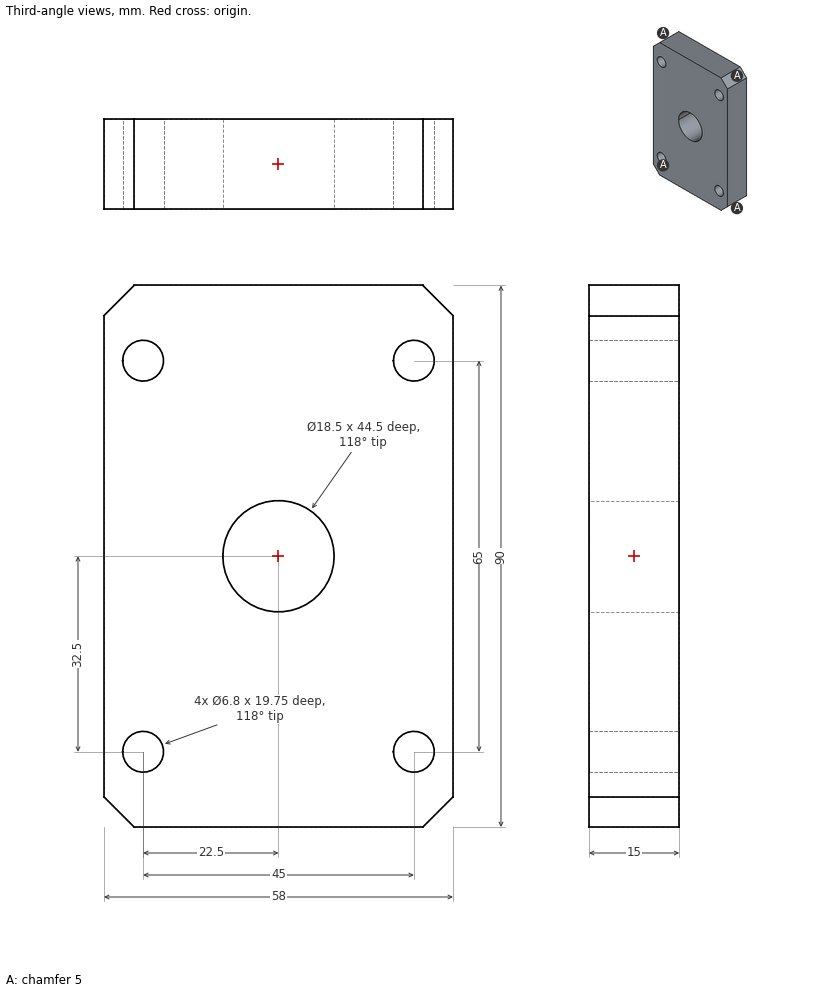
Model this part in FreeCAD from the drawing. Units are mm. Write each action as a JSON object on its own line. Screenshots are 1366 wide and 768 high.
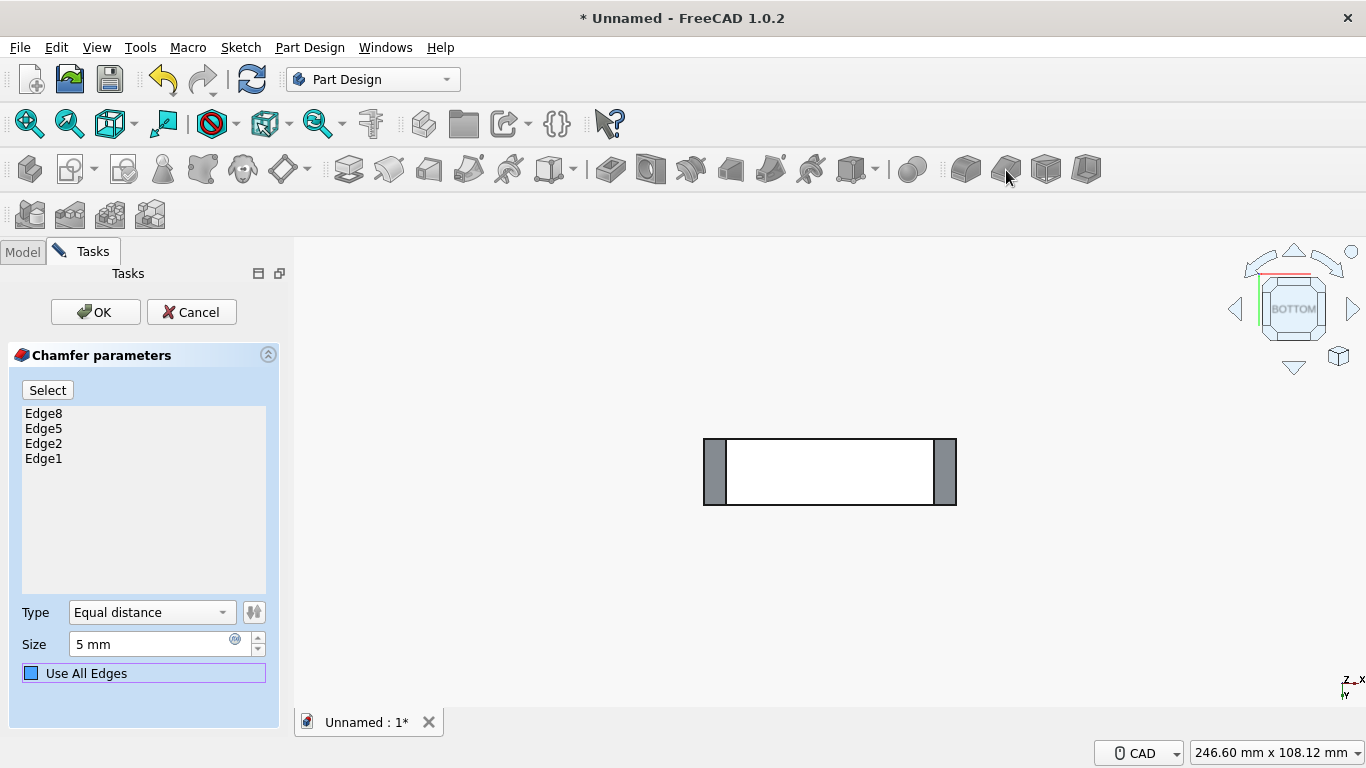
{"action": "left_click", "coordinate": [96, 312]}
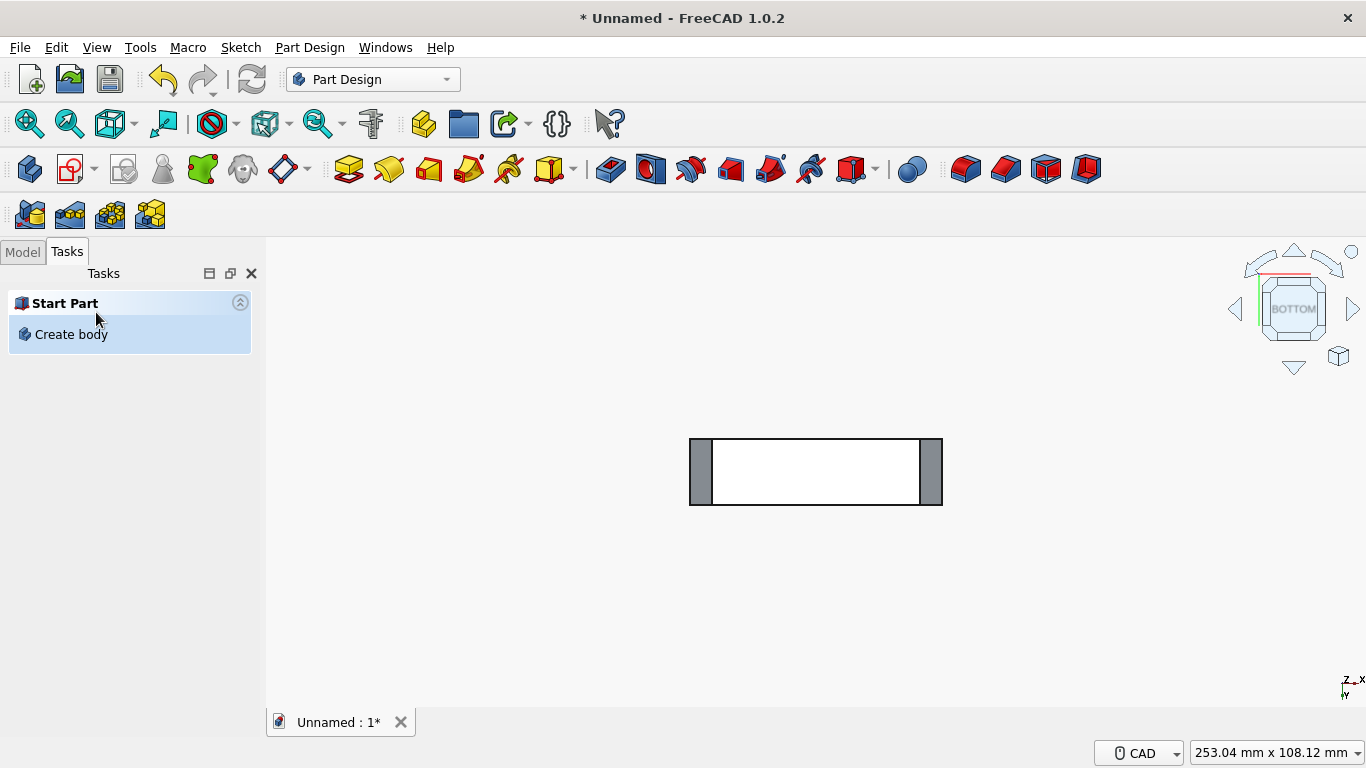
{"action": "key", "text": "0"}